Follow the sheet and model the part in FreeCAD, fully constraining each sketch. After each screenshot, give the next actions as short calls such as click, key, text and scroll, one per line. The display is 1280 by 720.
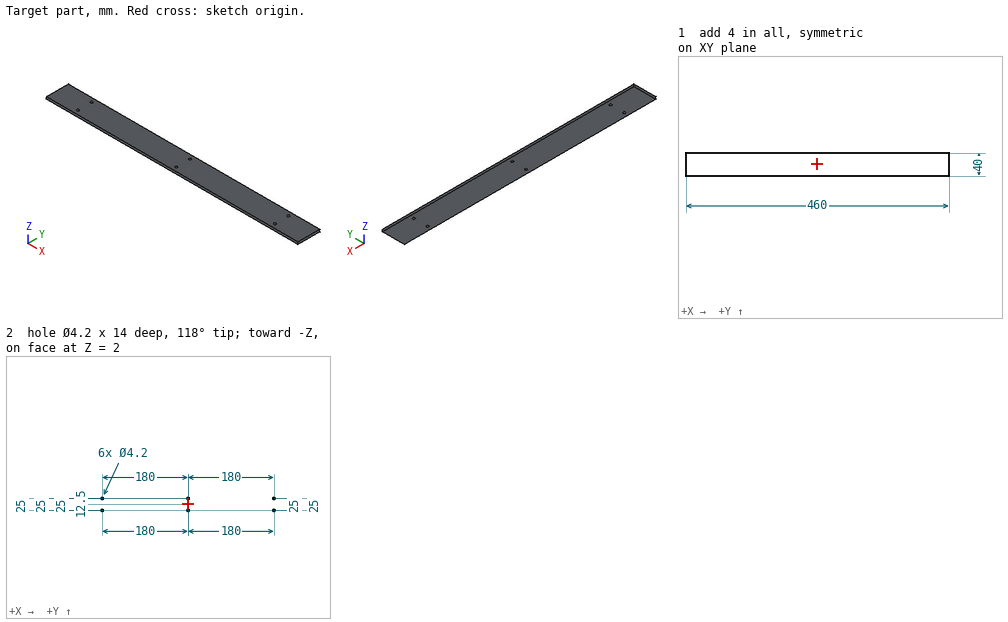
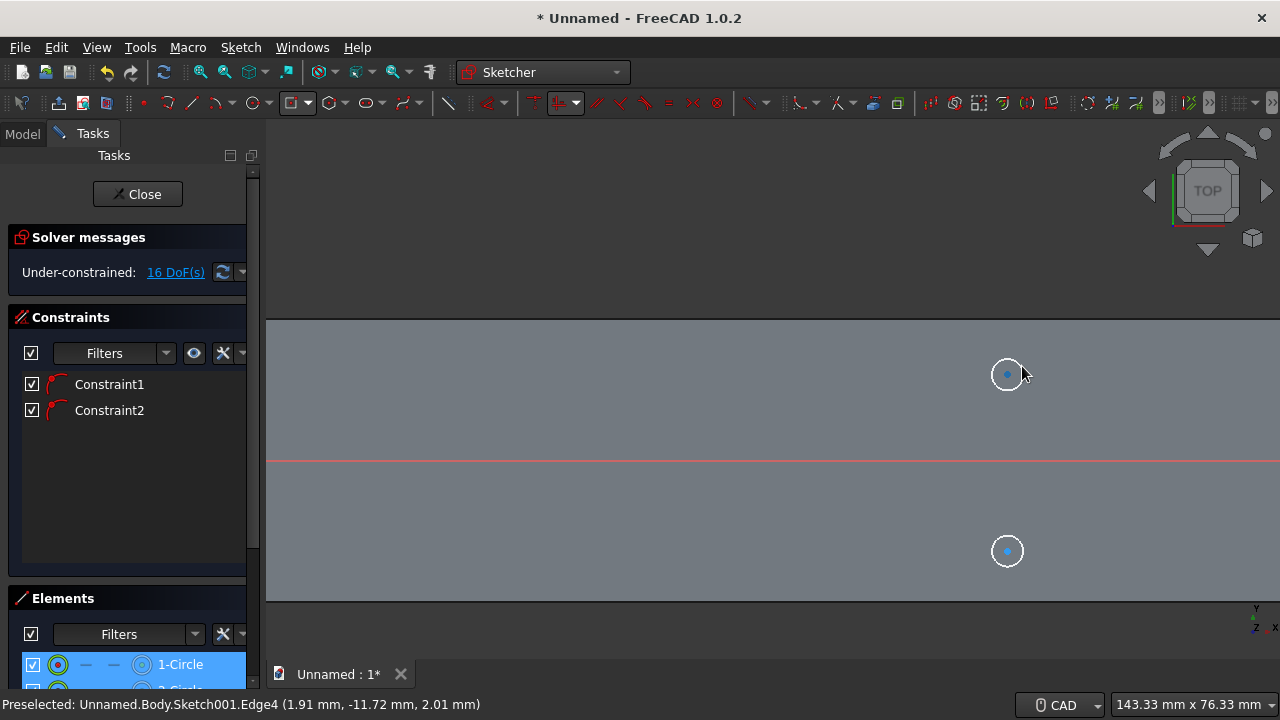
click(1019, 364)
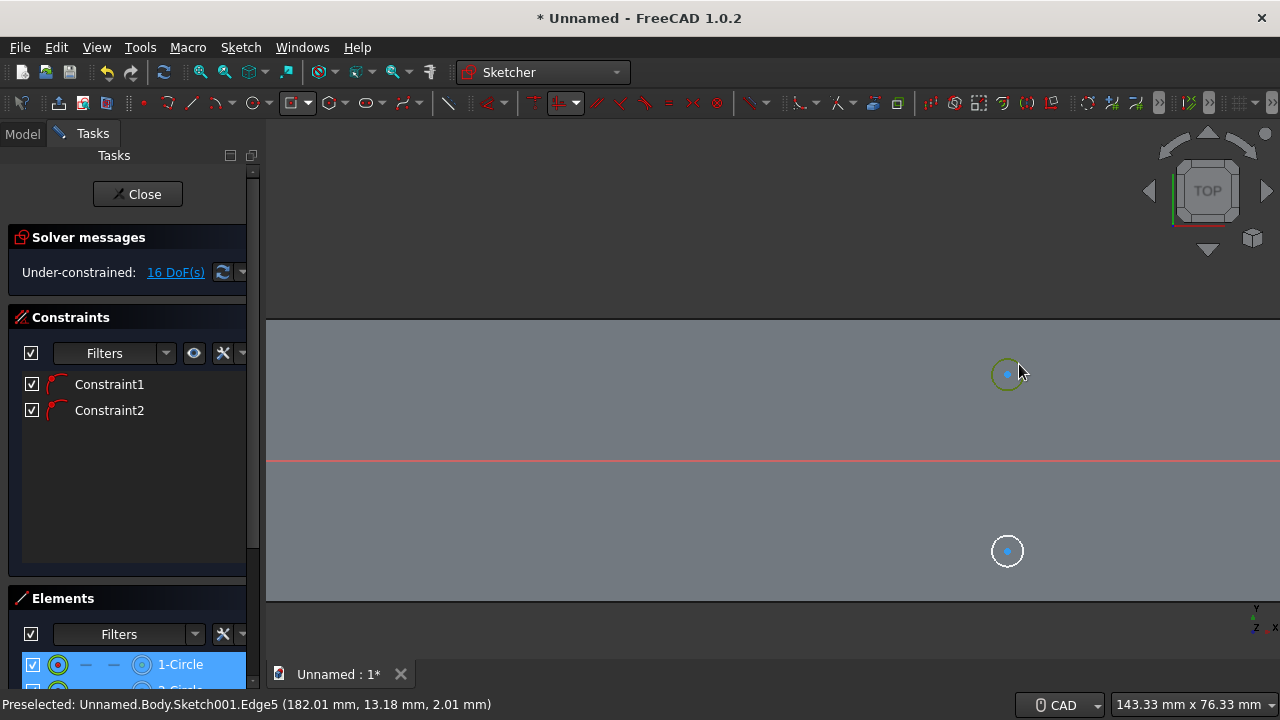
click(1018, 540)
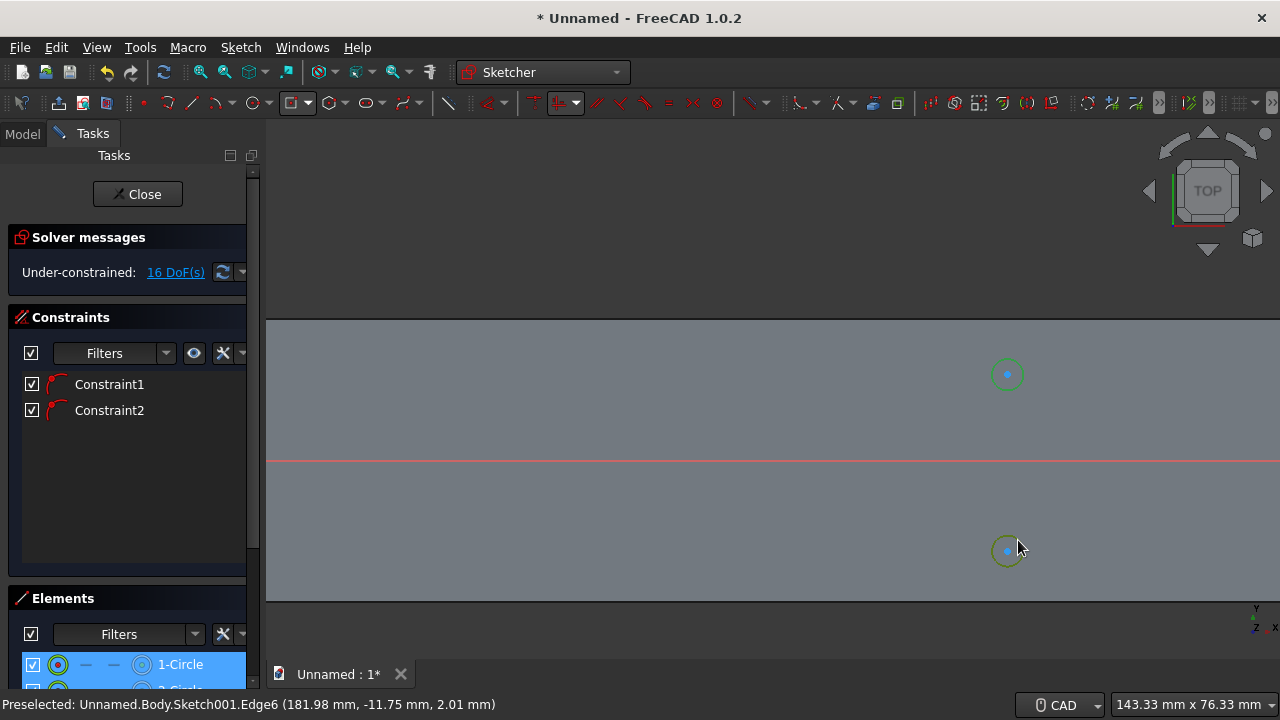
click(670, 104)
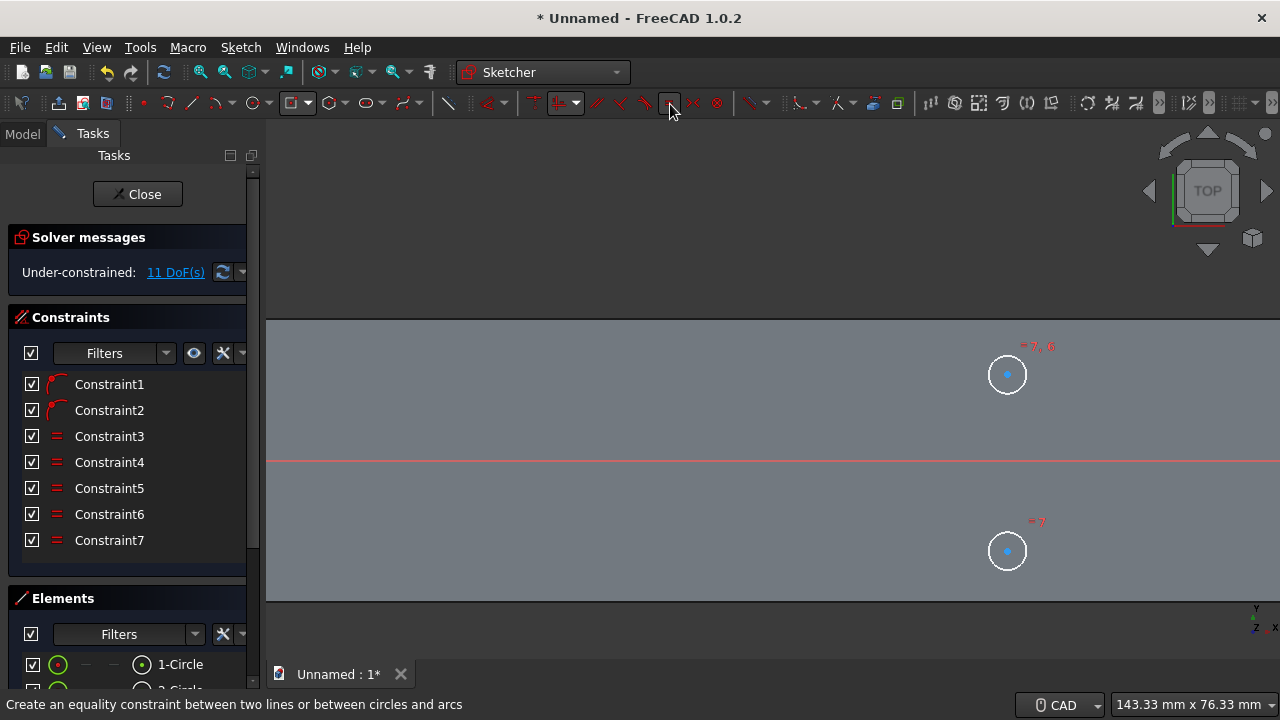
key(d)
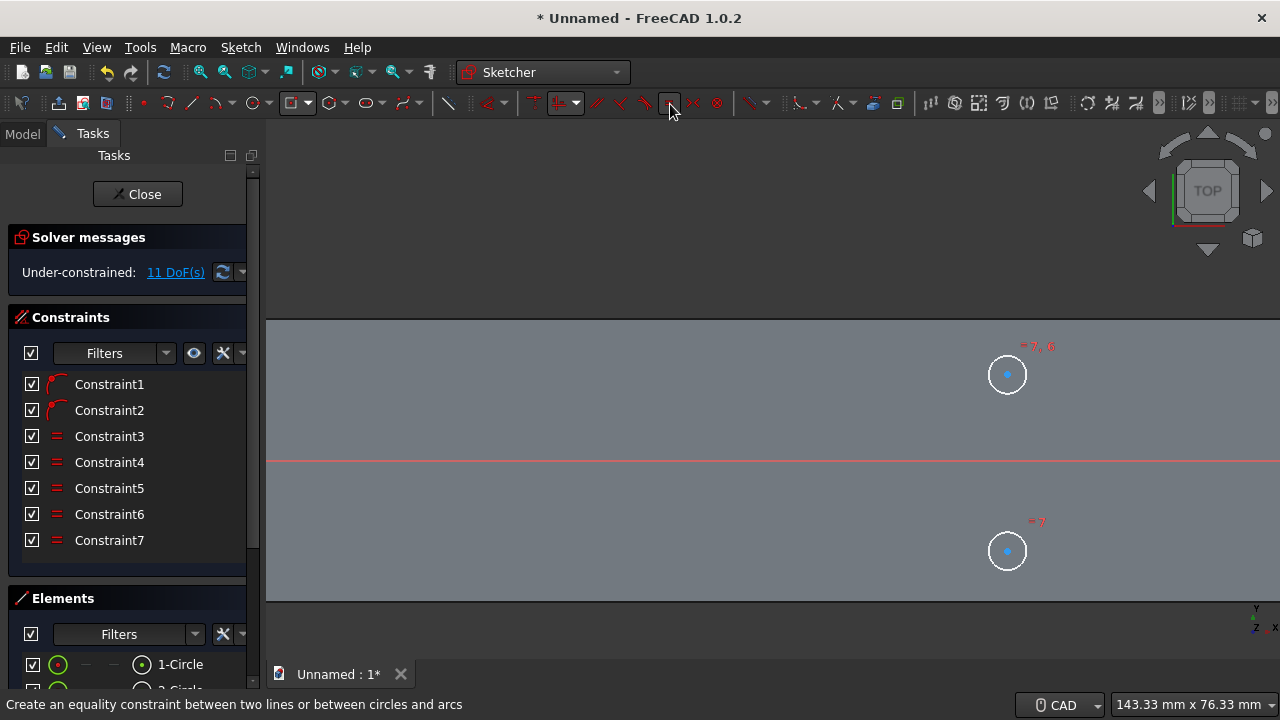
scroll(1022, 366, down, 7)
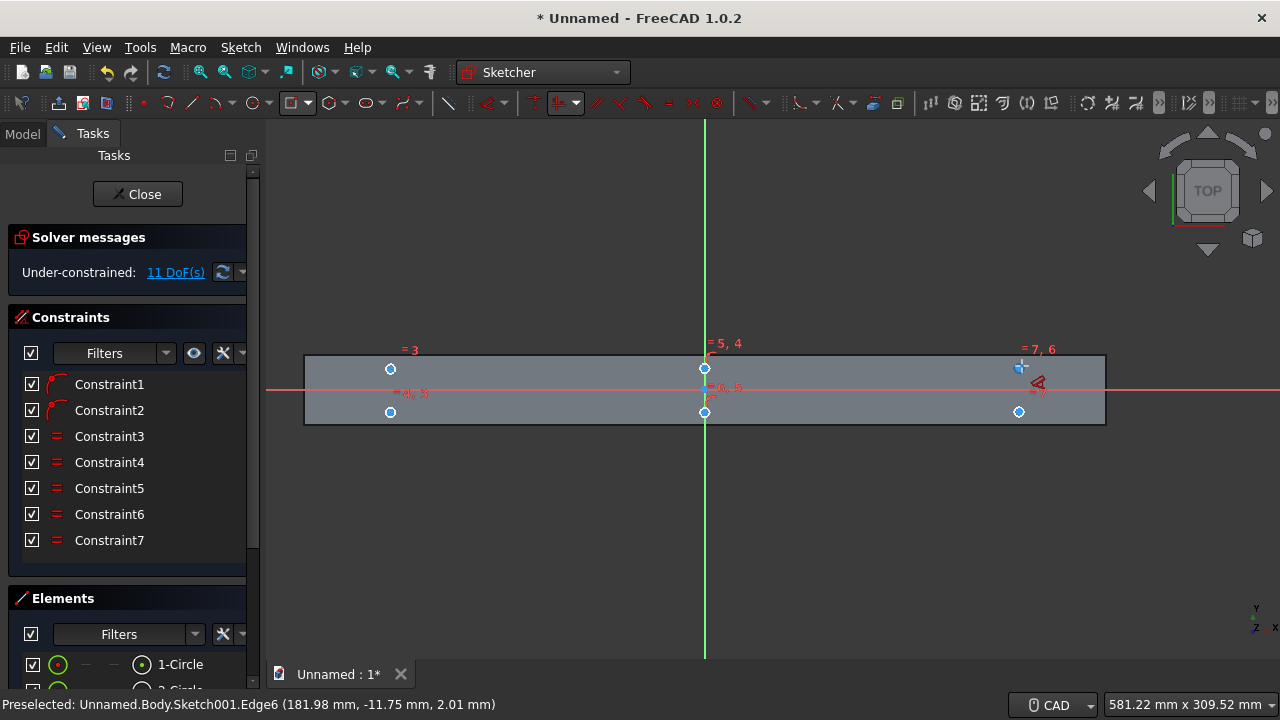
scroll(394, 366, up, 9)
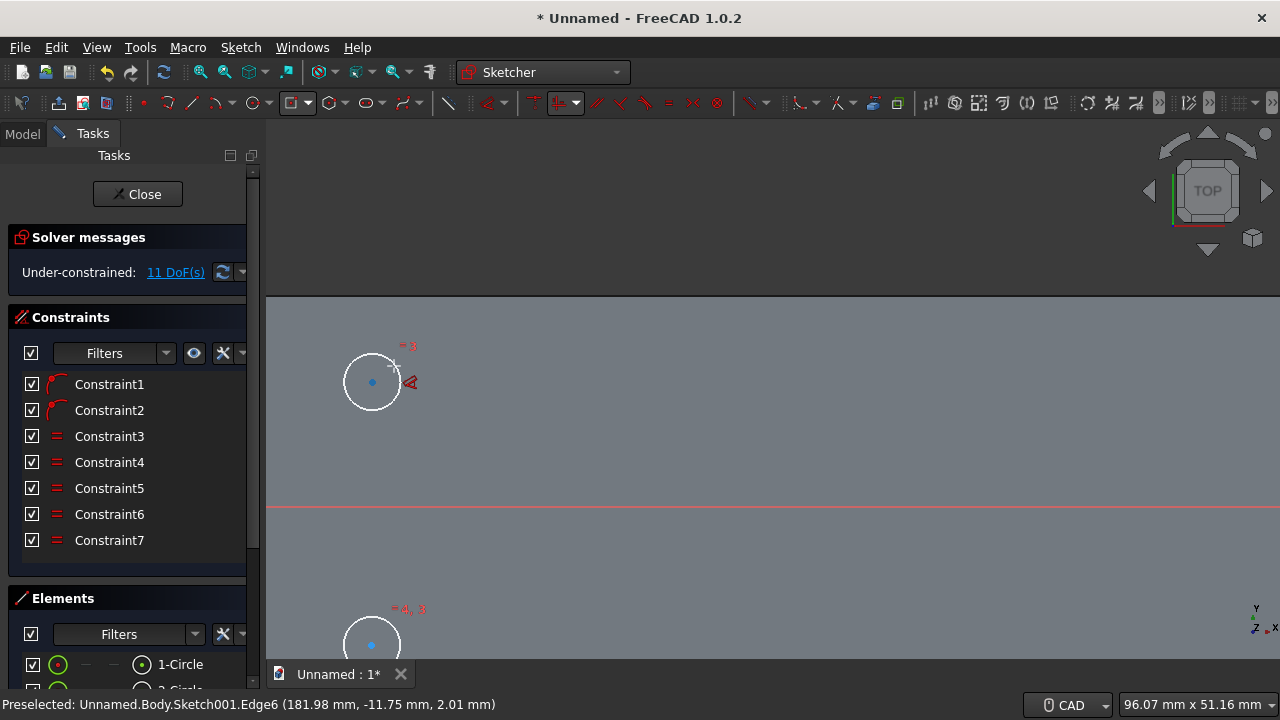
click(392, 362)
click(414, 339)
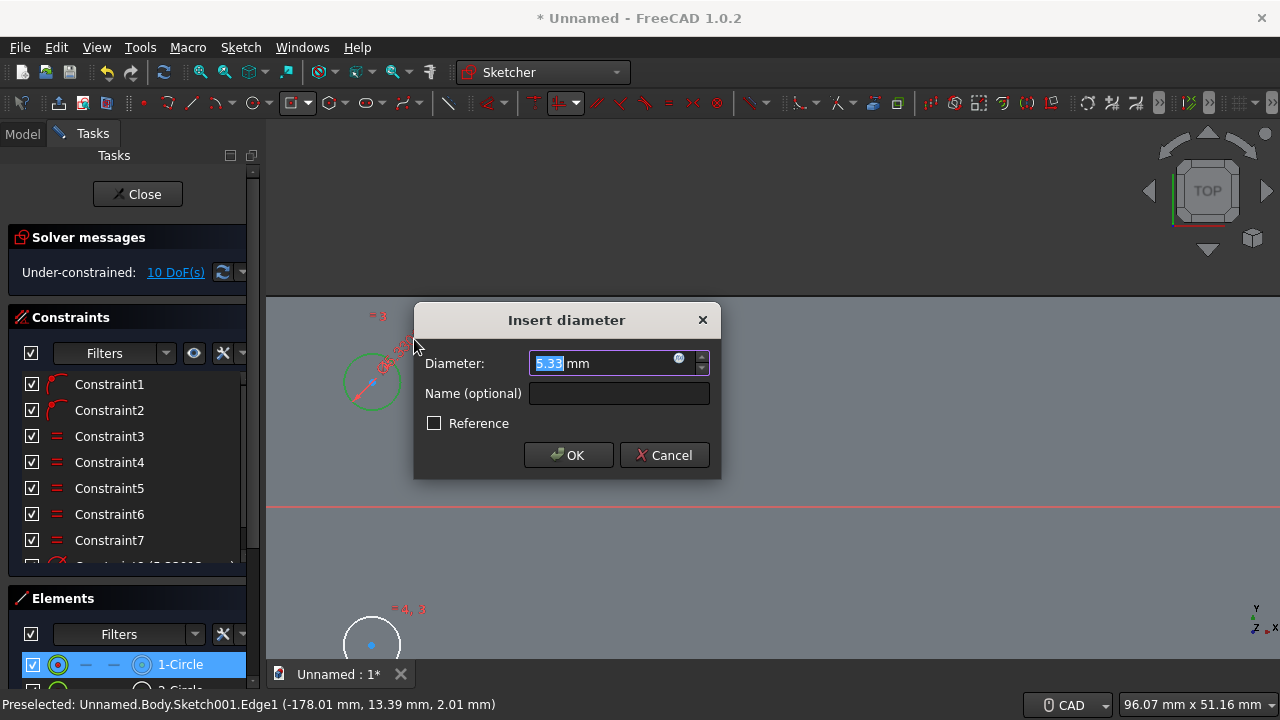
text(4.2)
key(Return)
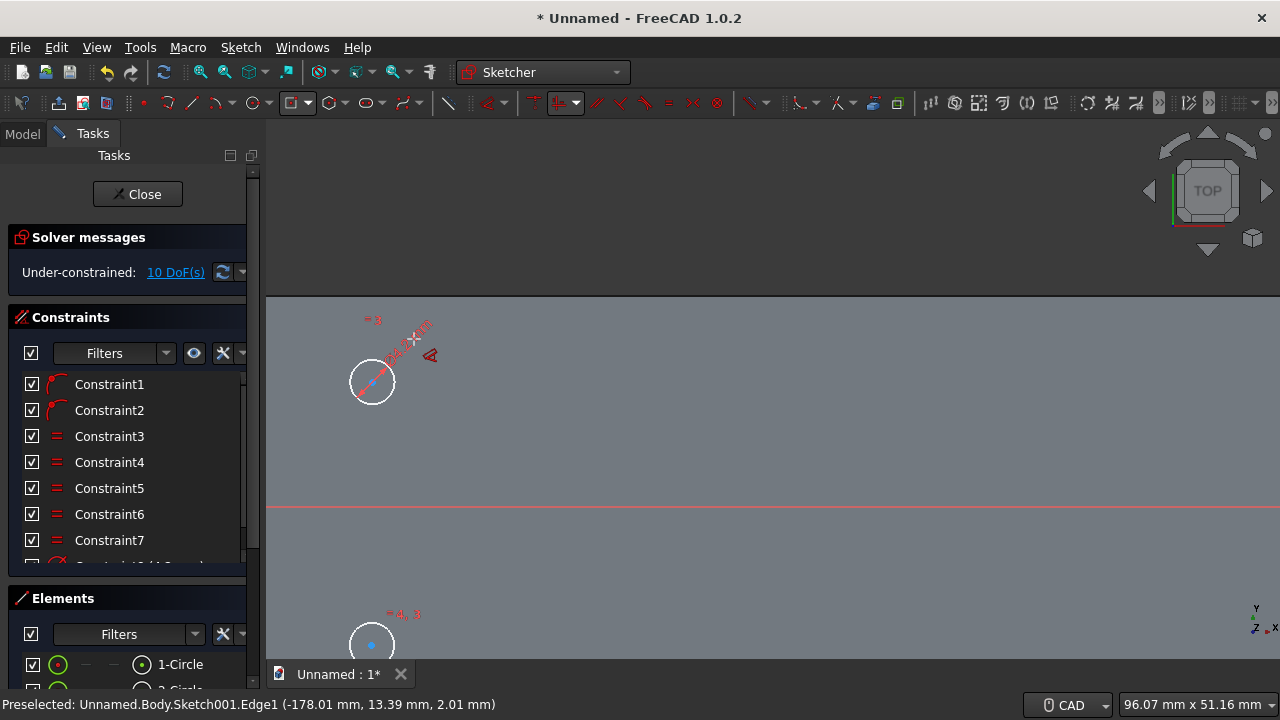
scroll(394, 366, down, 9)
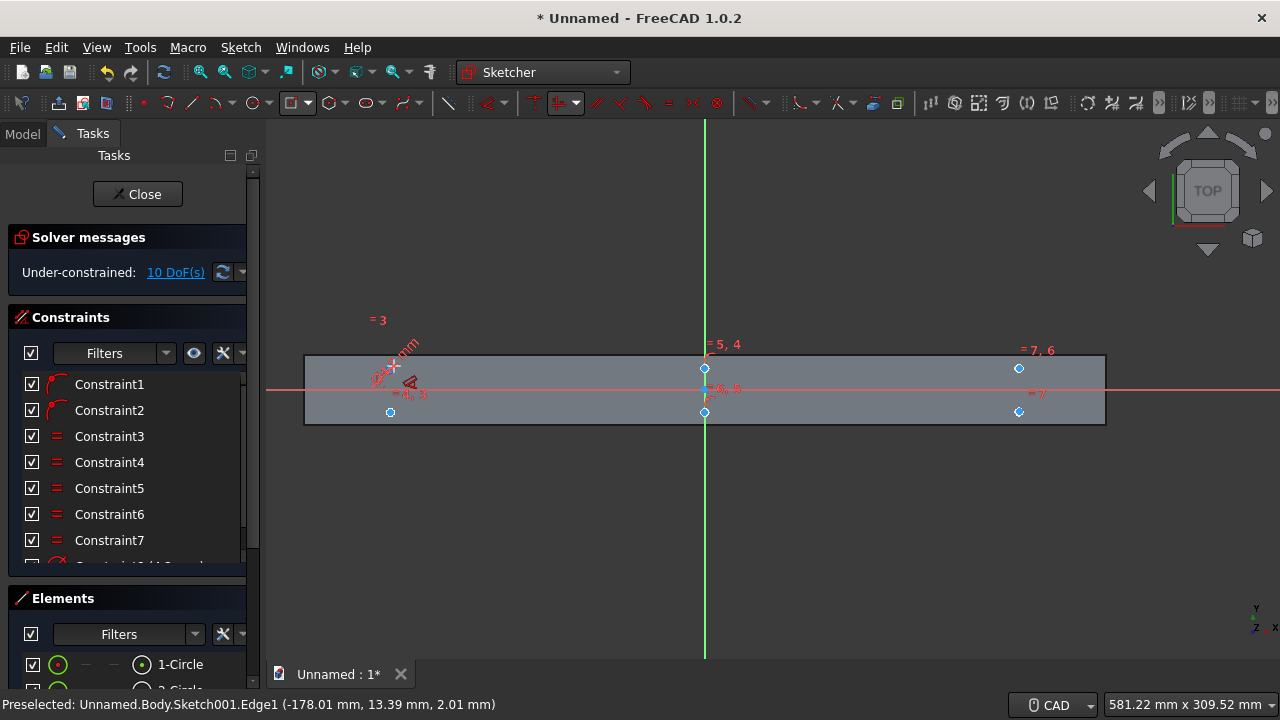
click(391, 369)
click(548, 335)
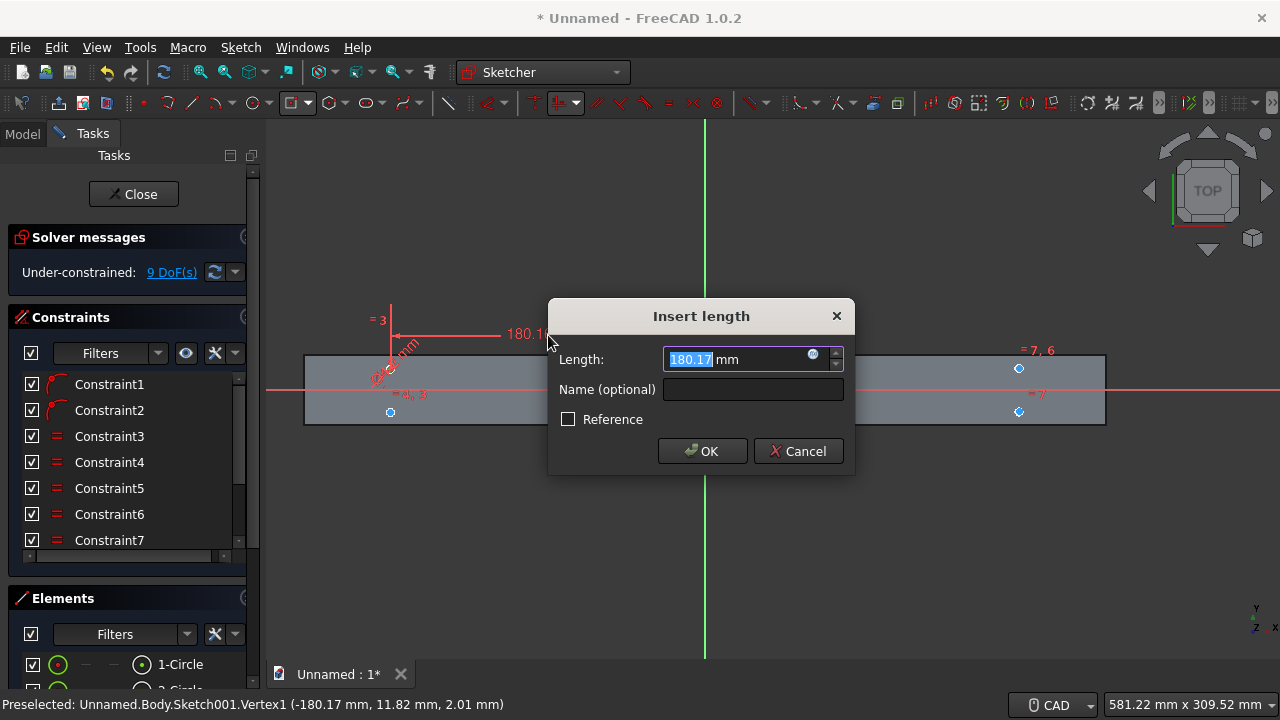
text(180)
key(Return)